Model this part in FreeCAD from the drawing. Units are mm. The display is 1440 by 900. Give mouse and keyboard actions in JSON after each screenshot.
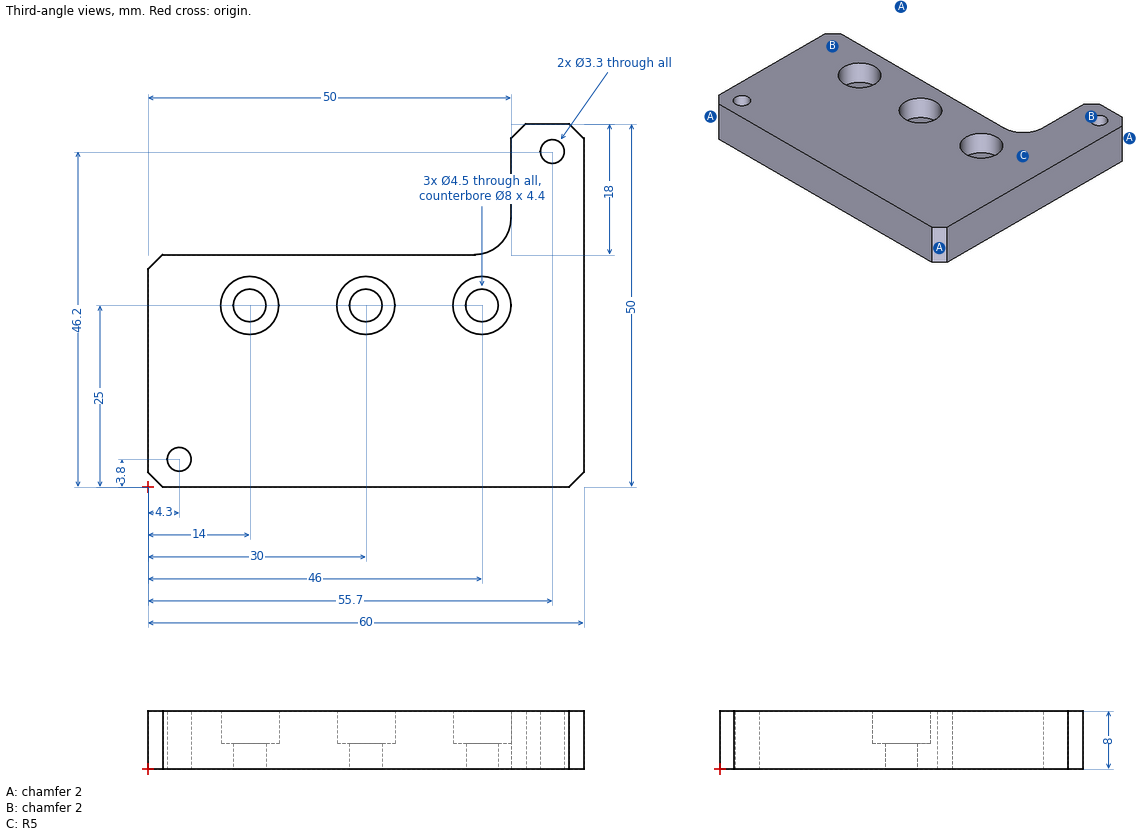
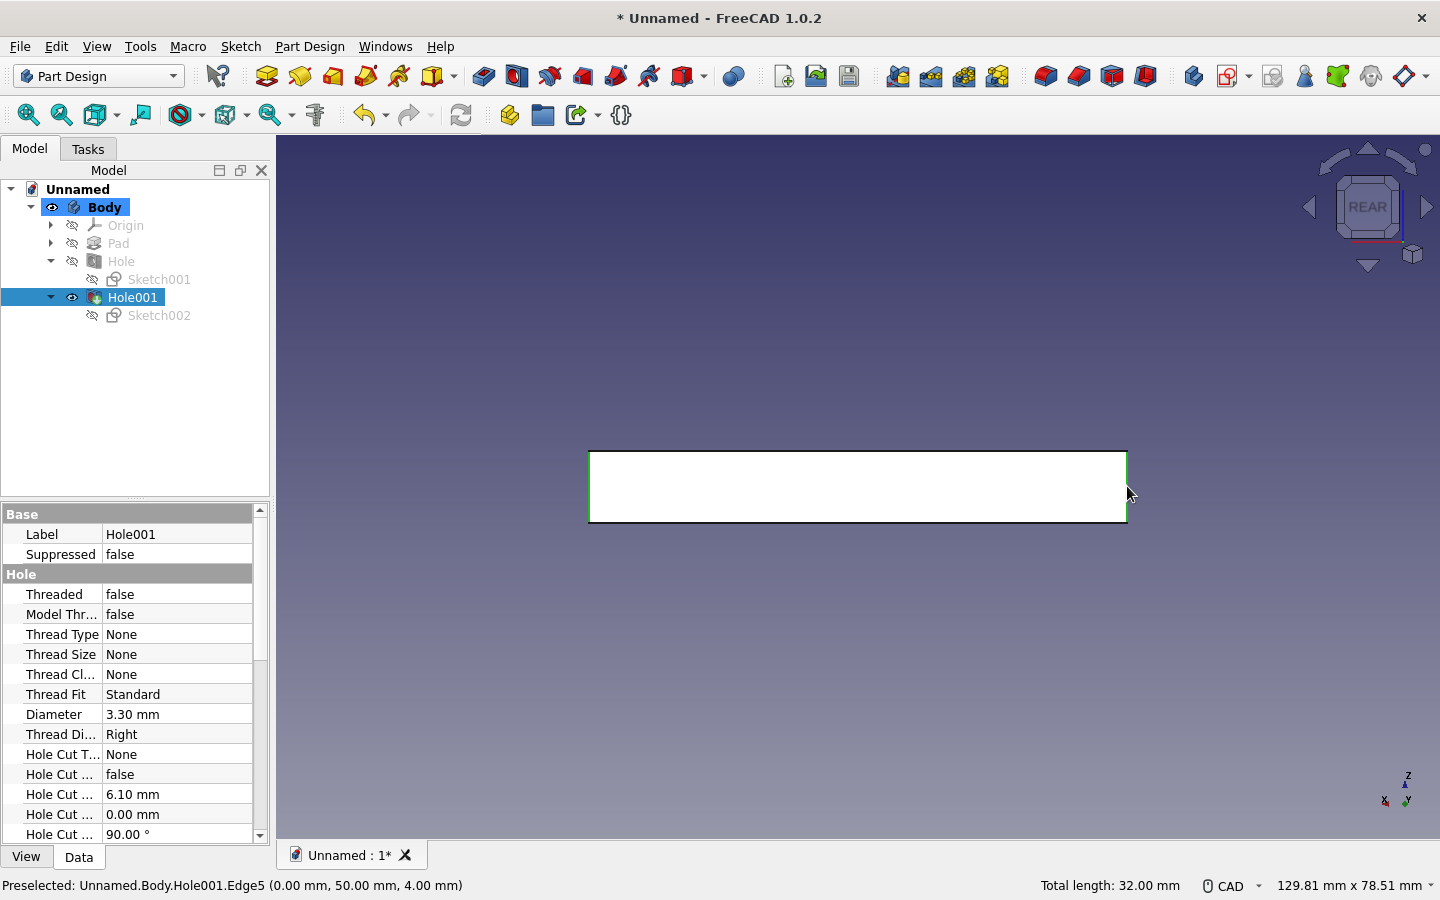
{"action": "left_click", "coordinate": [1079, 76]}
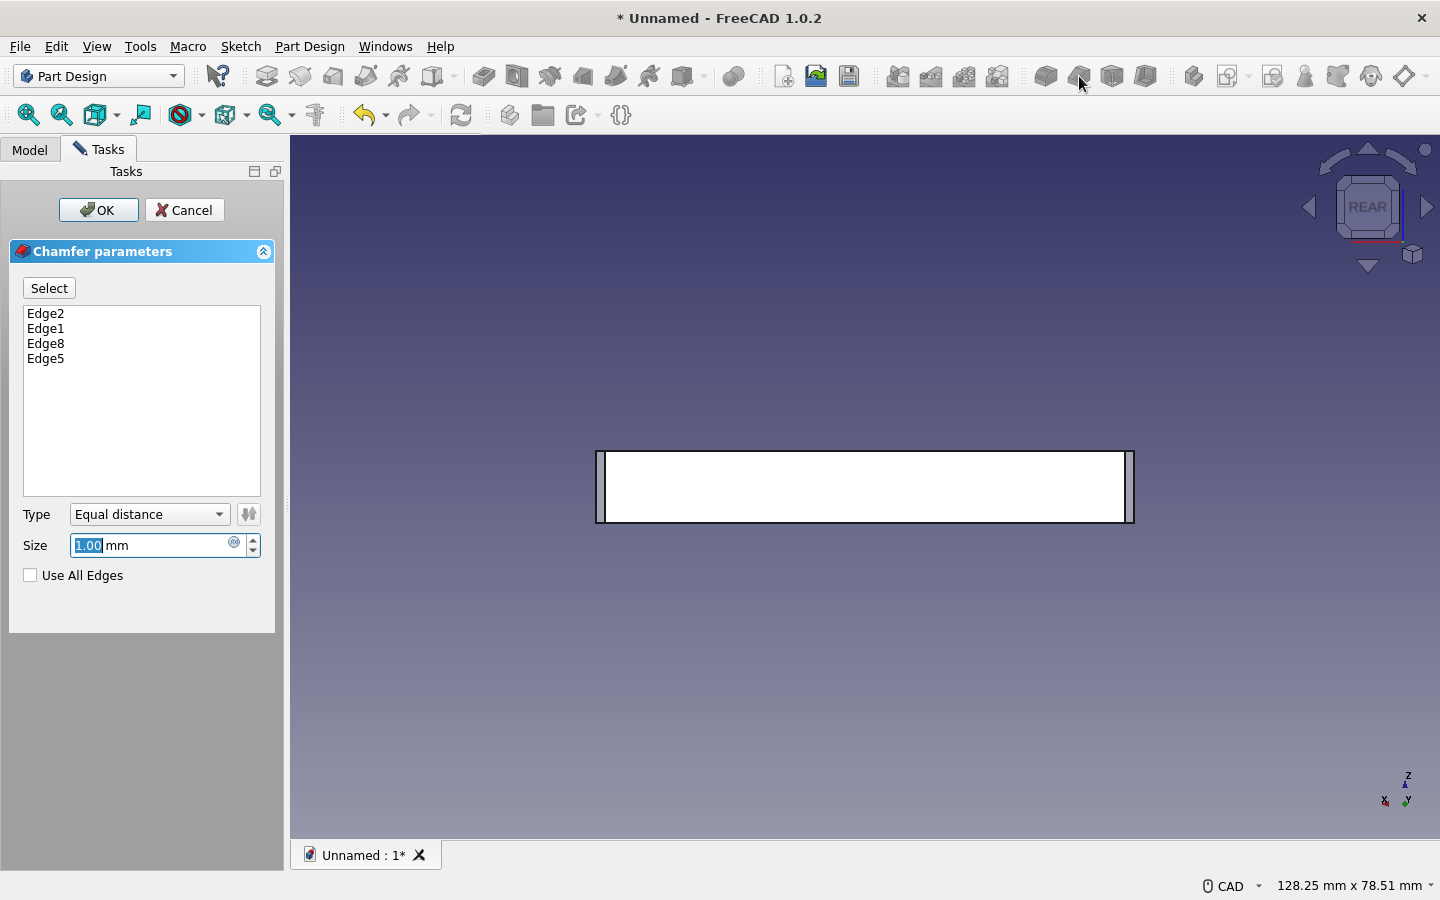
{"action": "type", "text": "2"}
{"action": "key", "text": "Tab"}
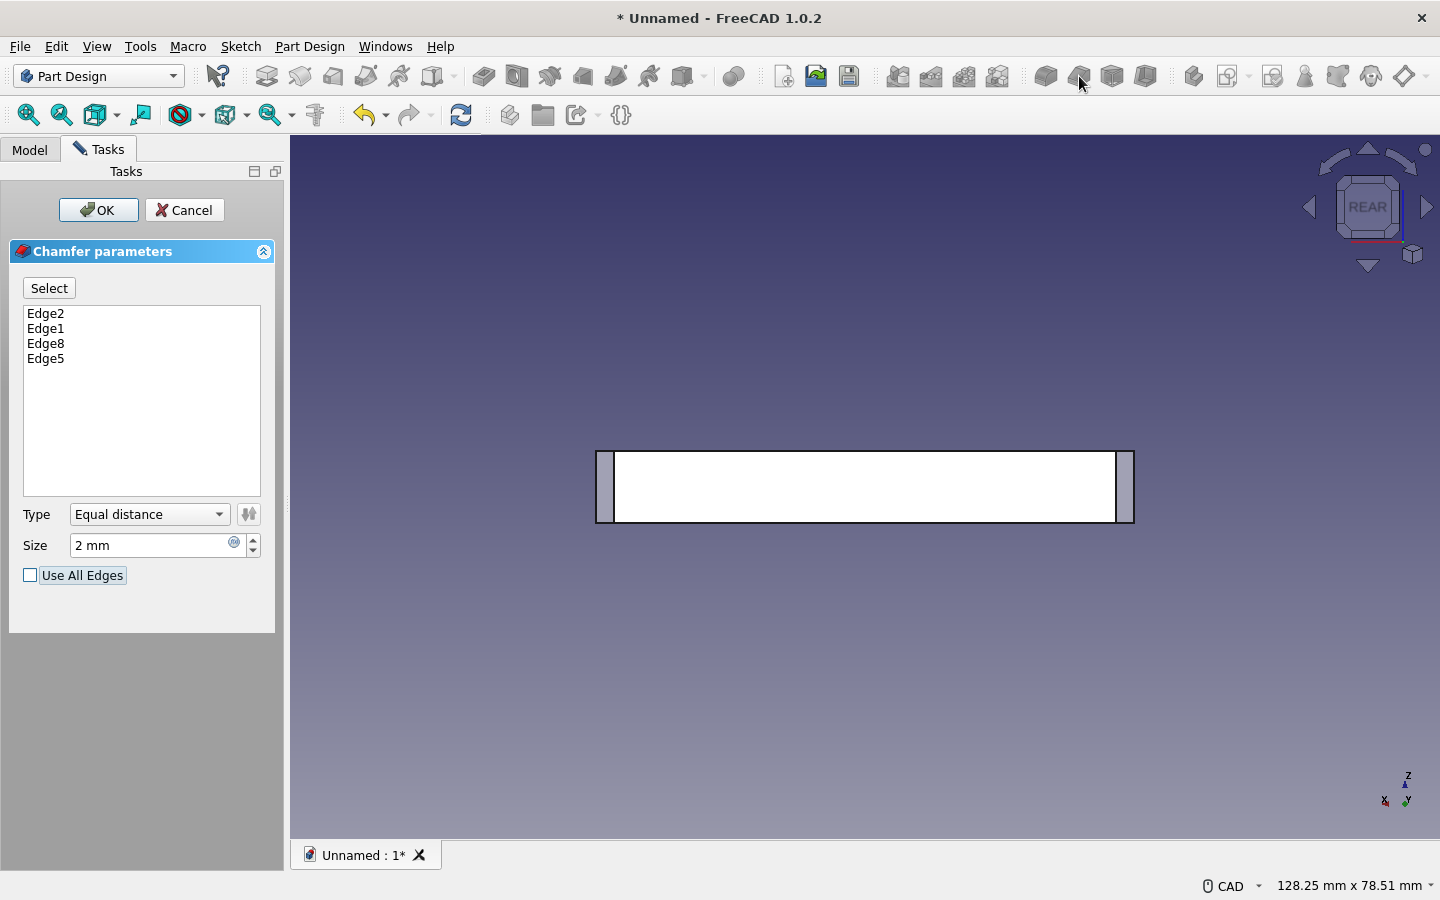
{"action": "left_click", "coordinate": [99, 210]}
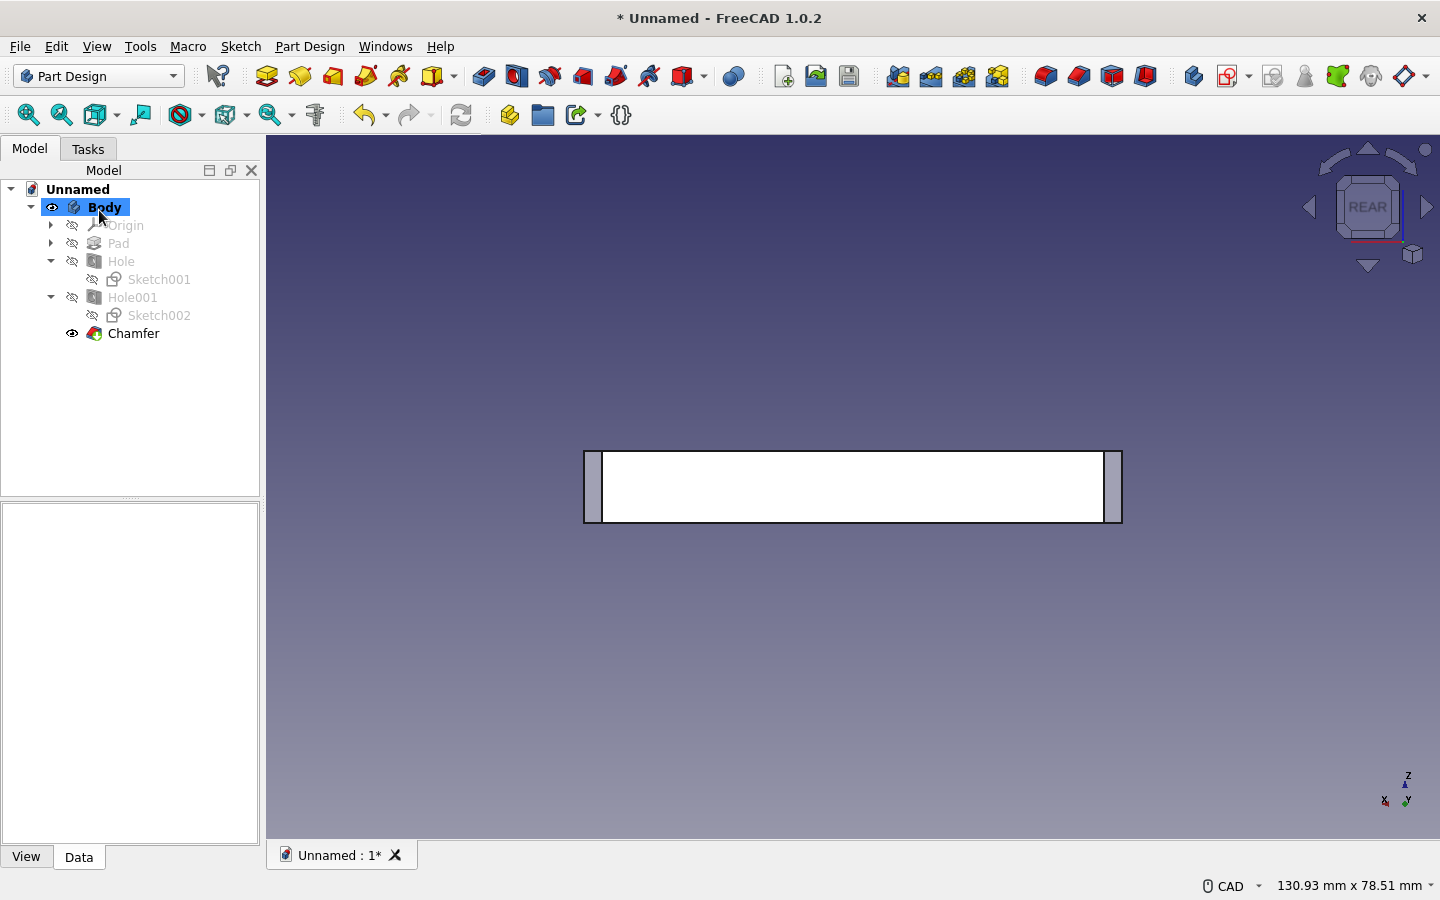
{"action": "left_click", "coordinate": [1226, 76]}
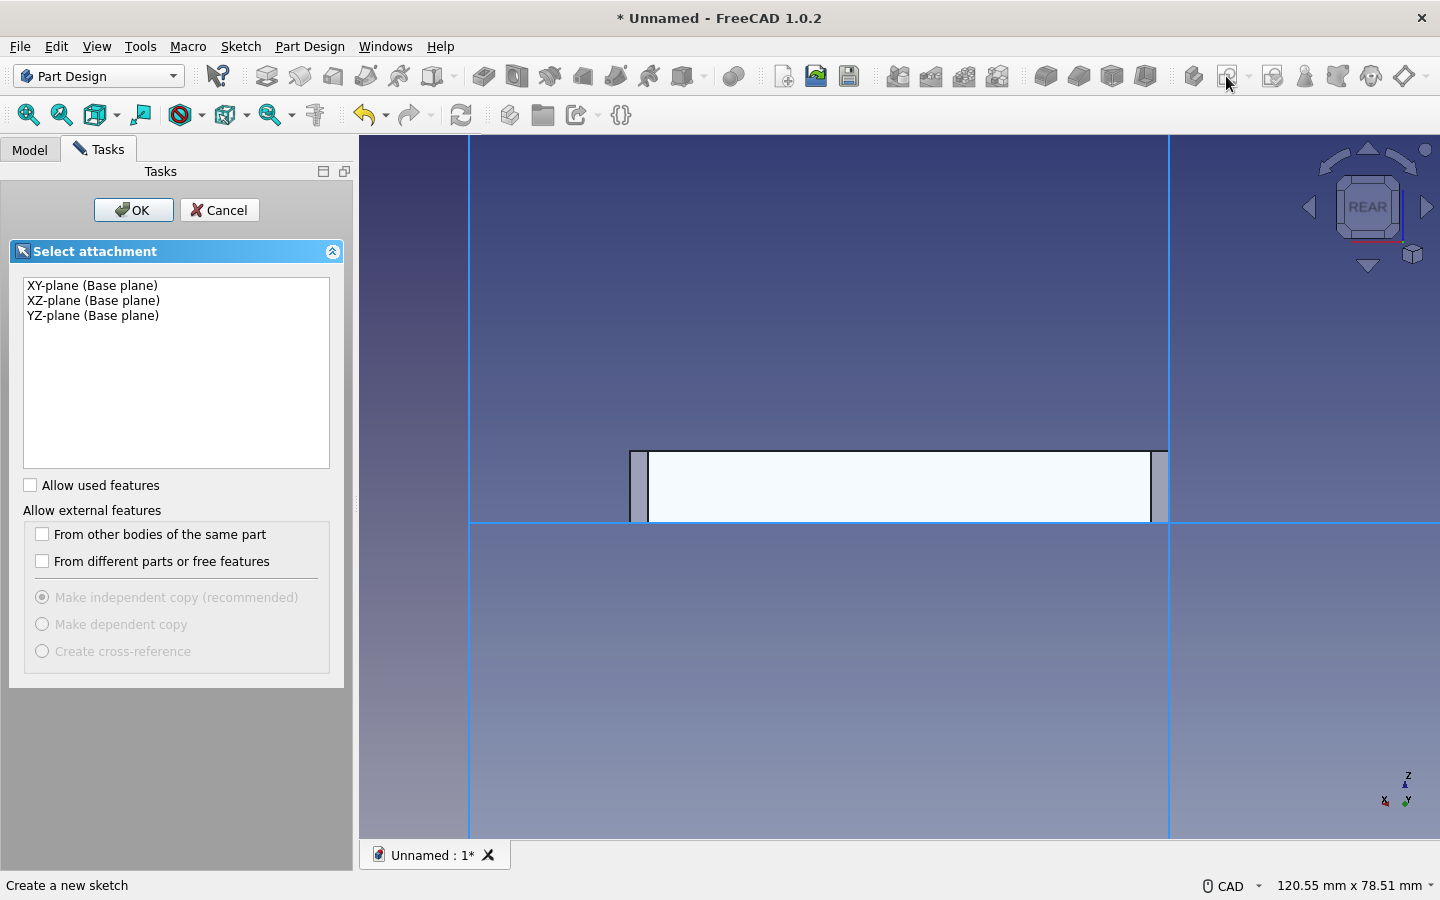
{"action": "left_click", "coordinate": [84, 286]}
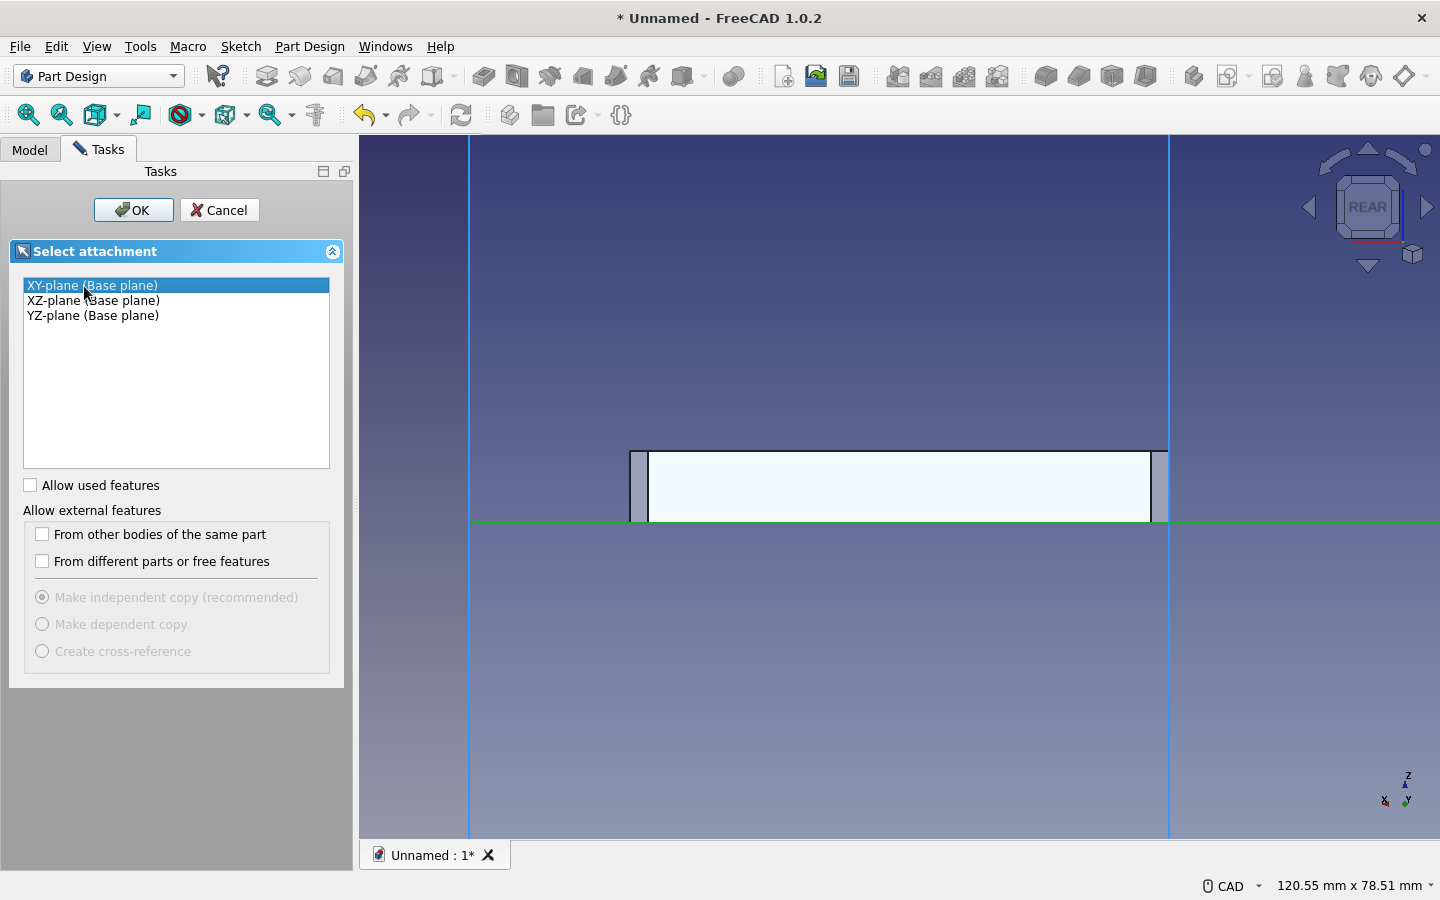
{"action": "left_click", "coordinate": [134, 210]}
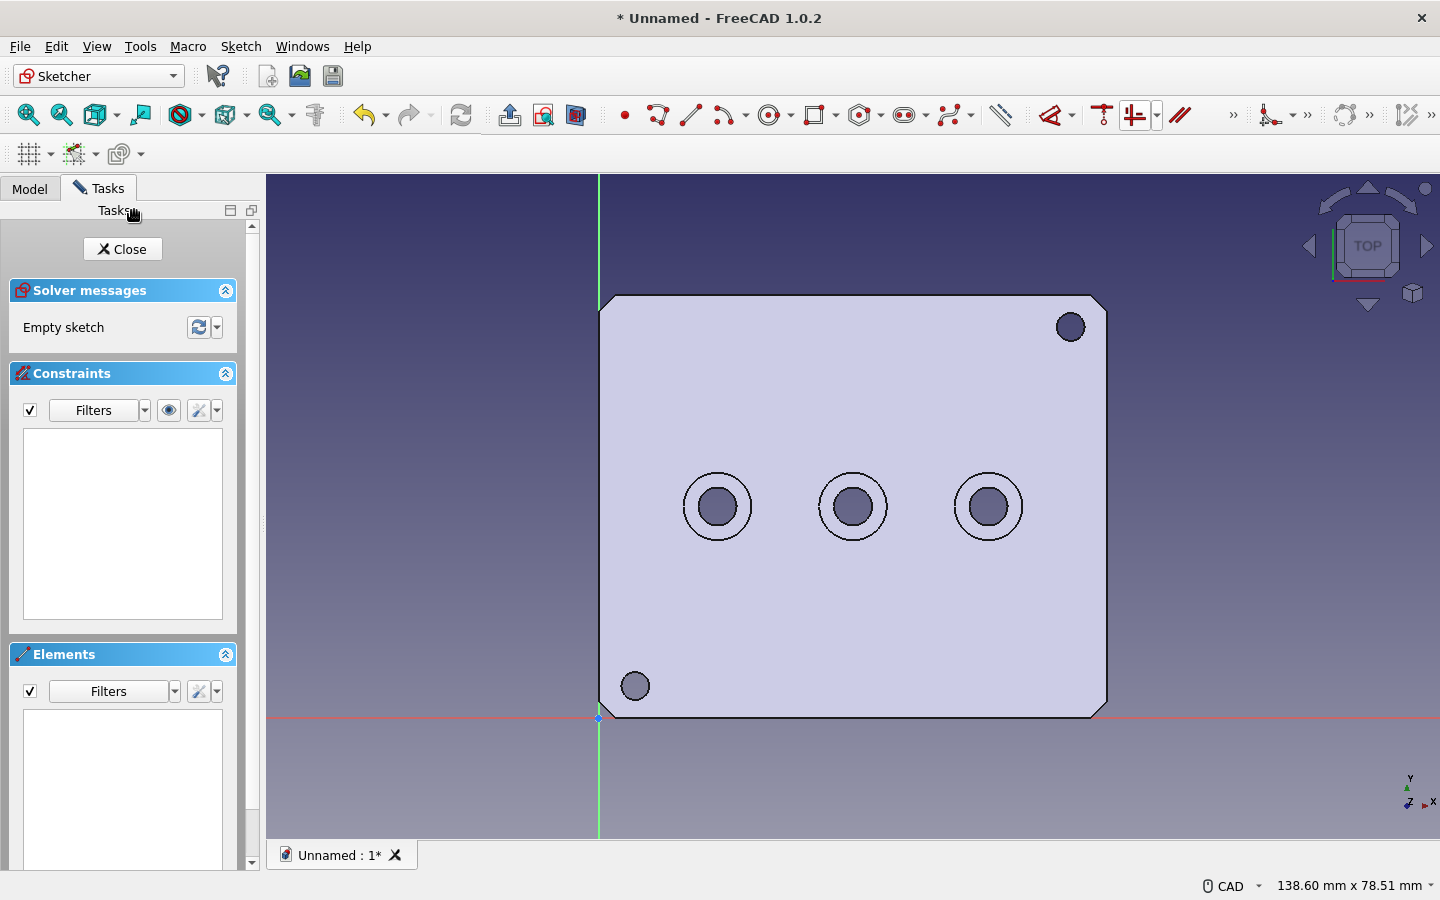
{"action": "left_click", "coordinate": [576, 116]}